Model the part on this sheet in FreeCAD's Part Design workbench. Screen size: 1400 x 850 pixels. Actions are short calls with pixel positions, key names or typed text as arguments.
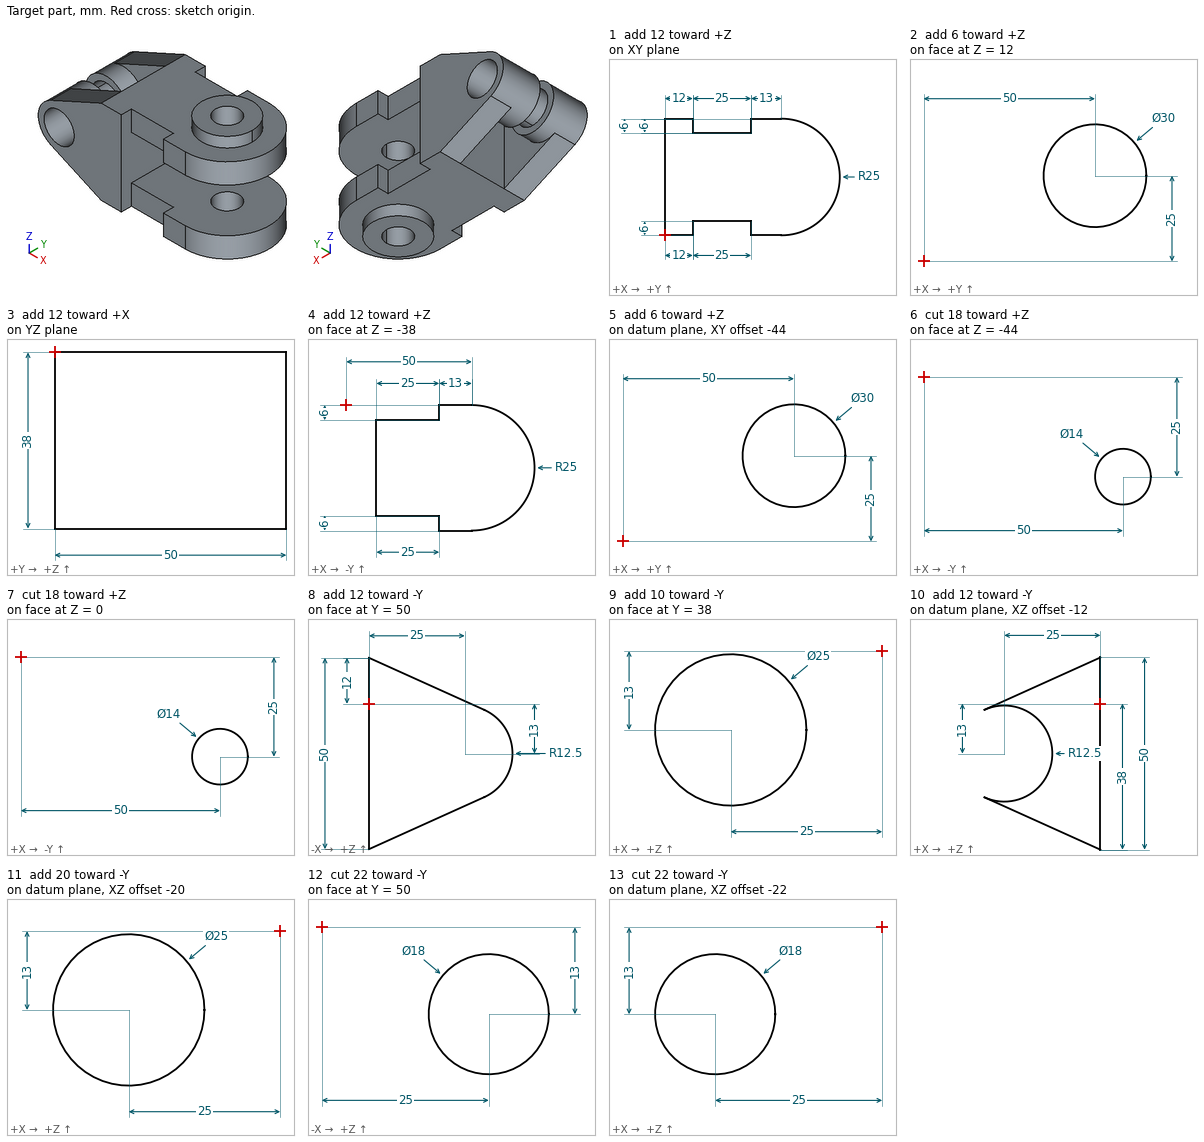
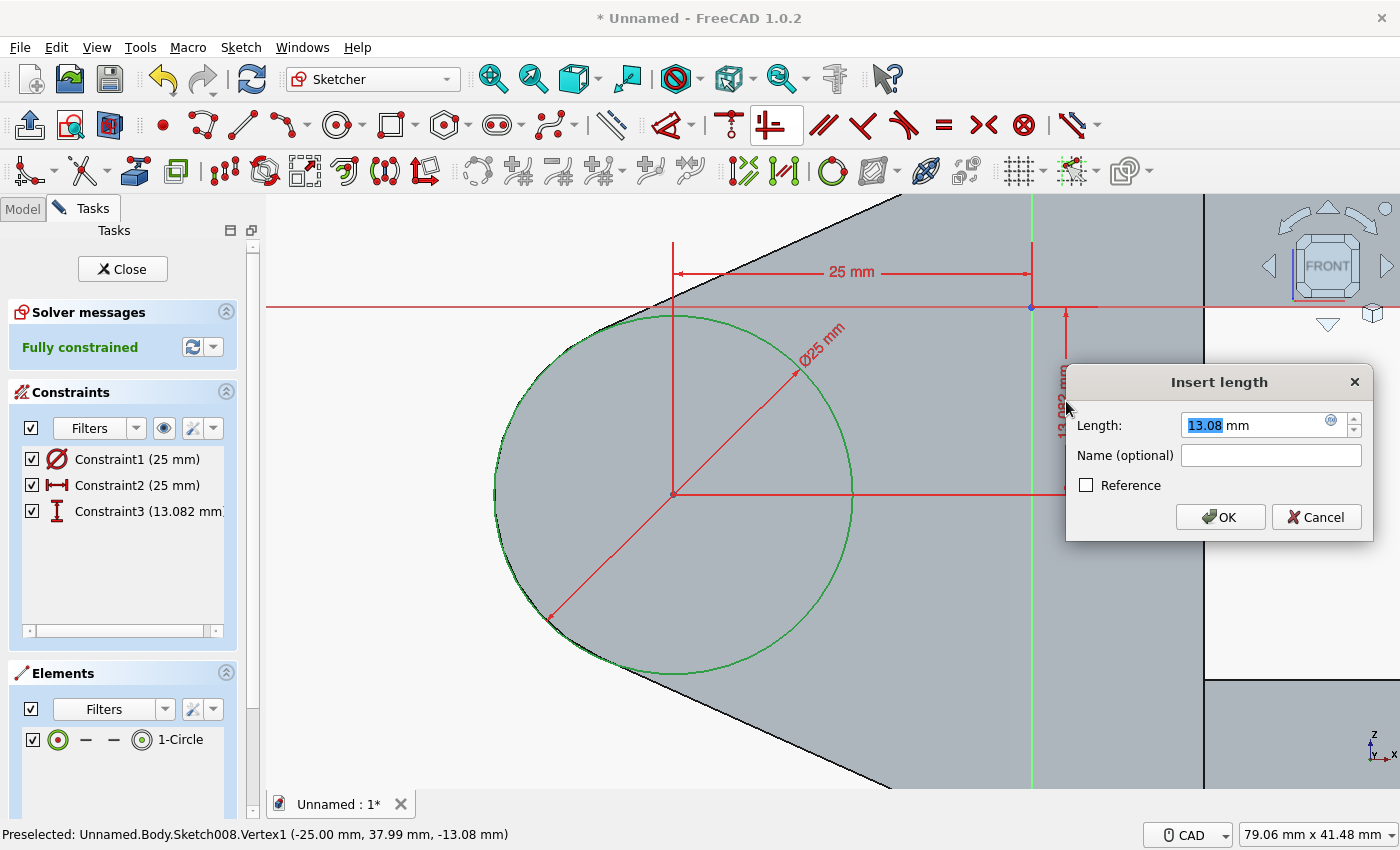
text(13)
key(Return)
key(Escape)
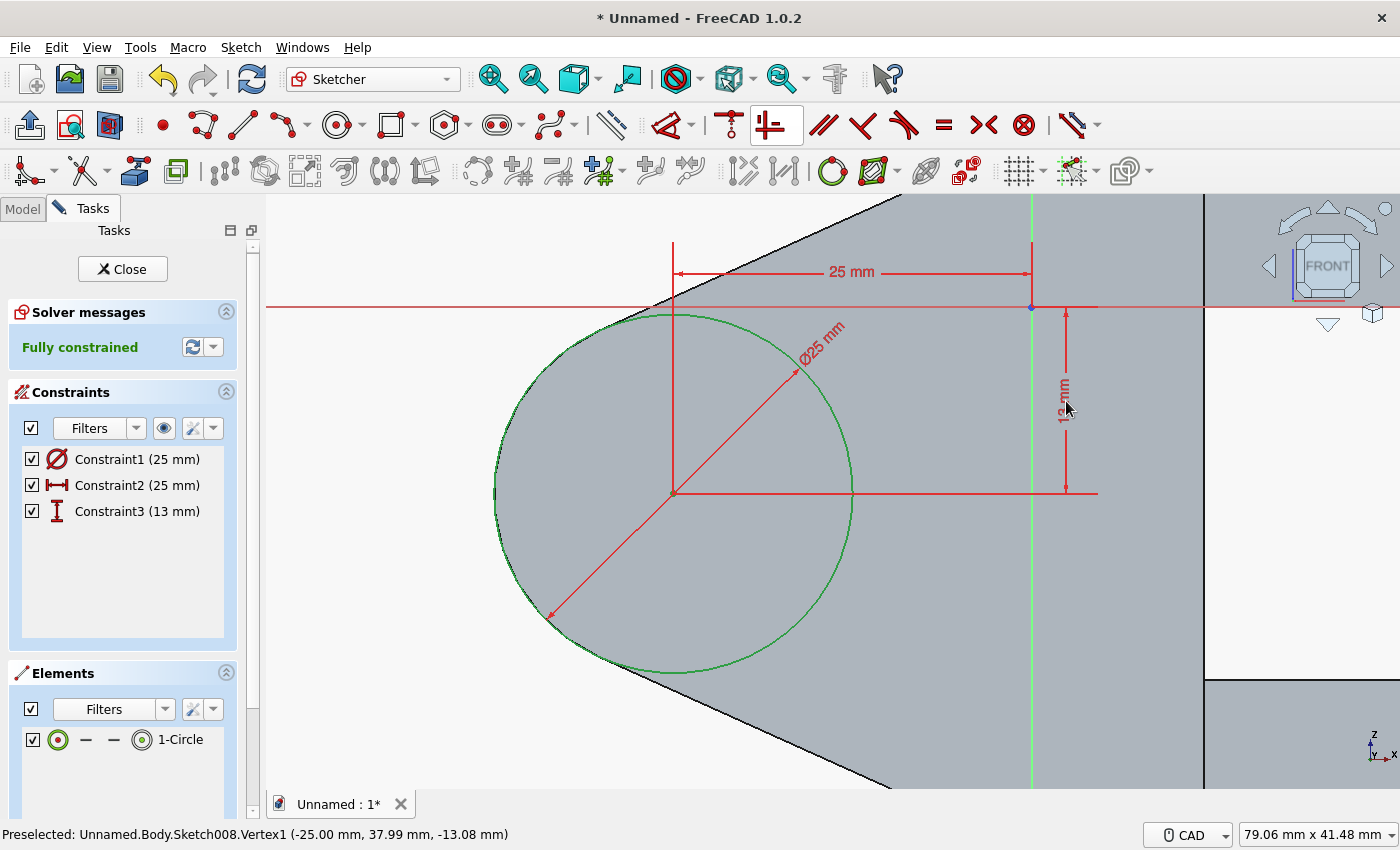
click(123, 269)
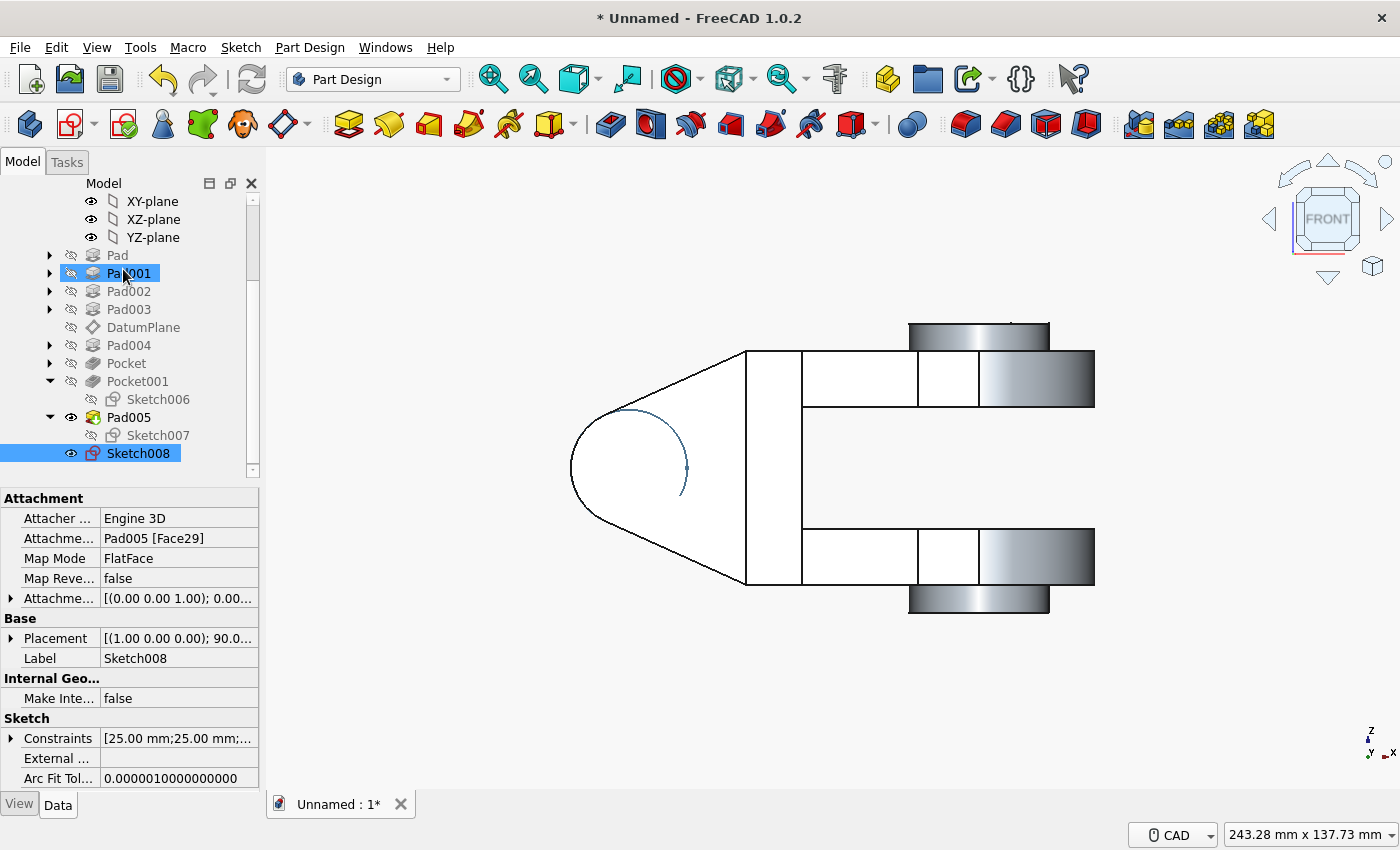
click(350, 124)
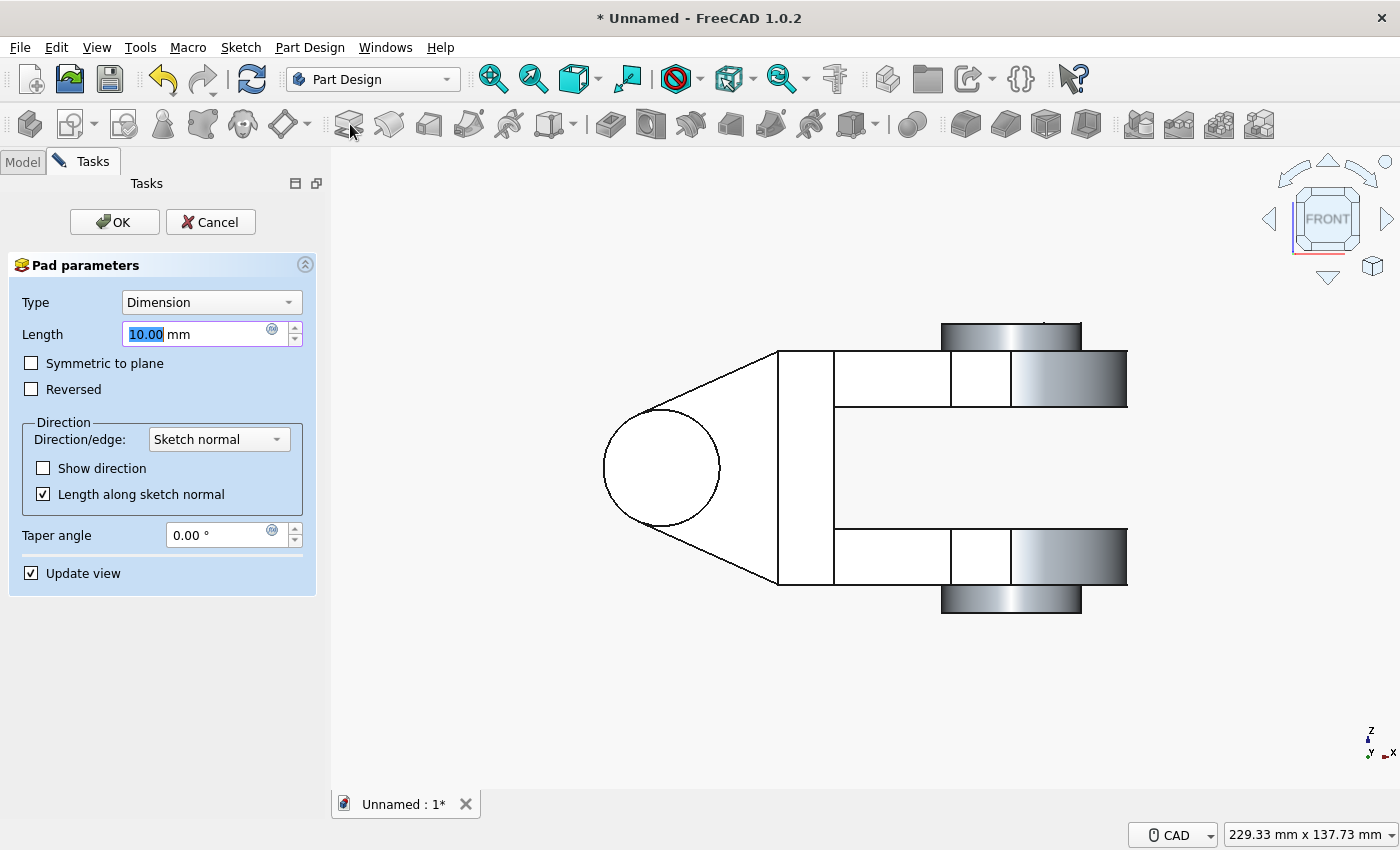
text(10)
key(Tab)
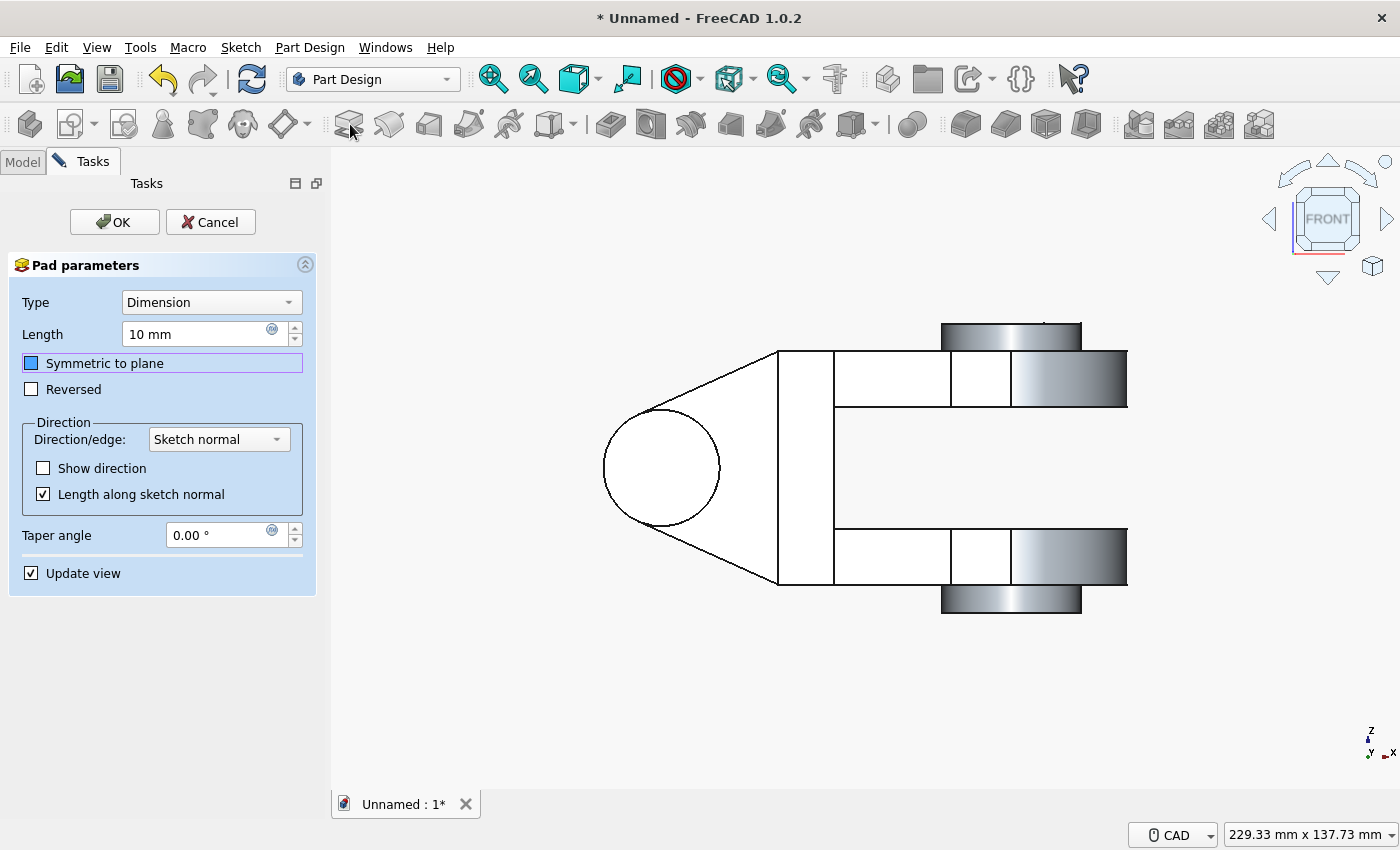
click(115, 222)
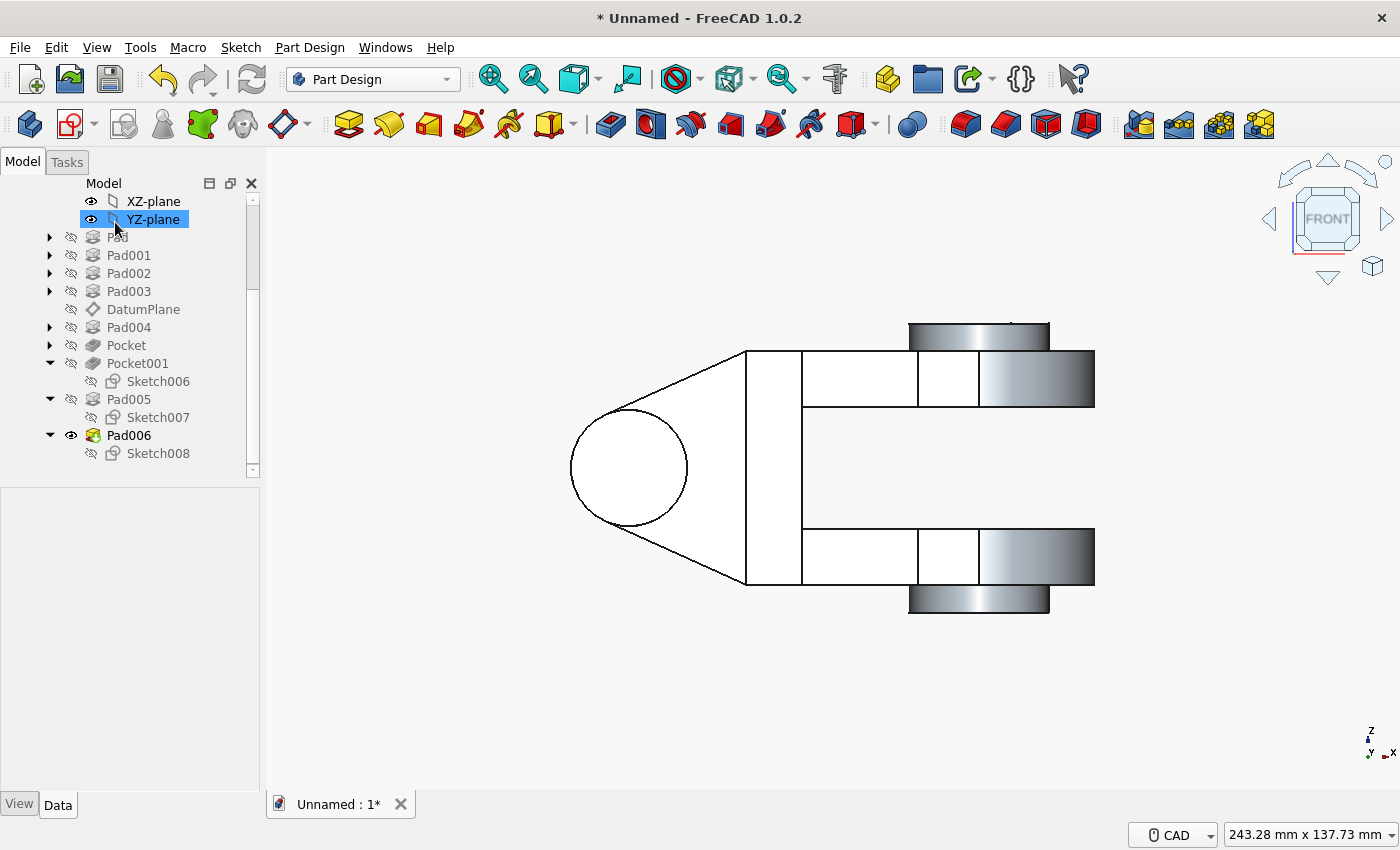
scroll(160, 323, down, 3)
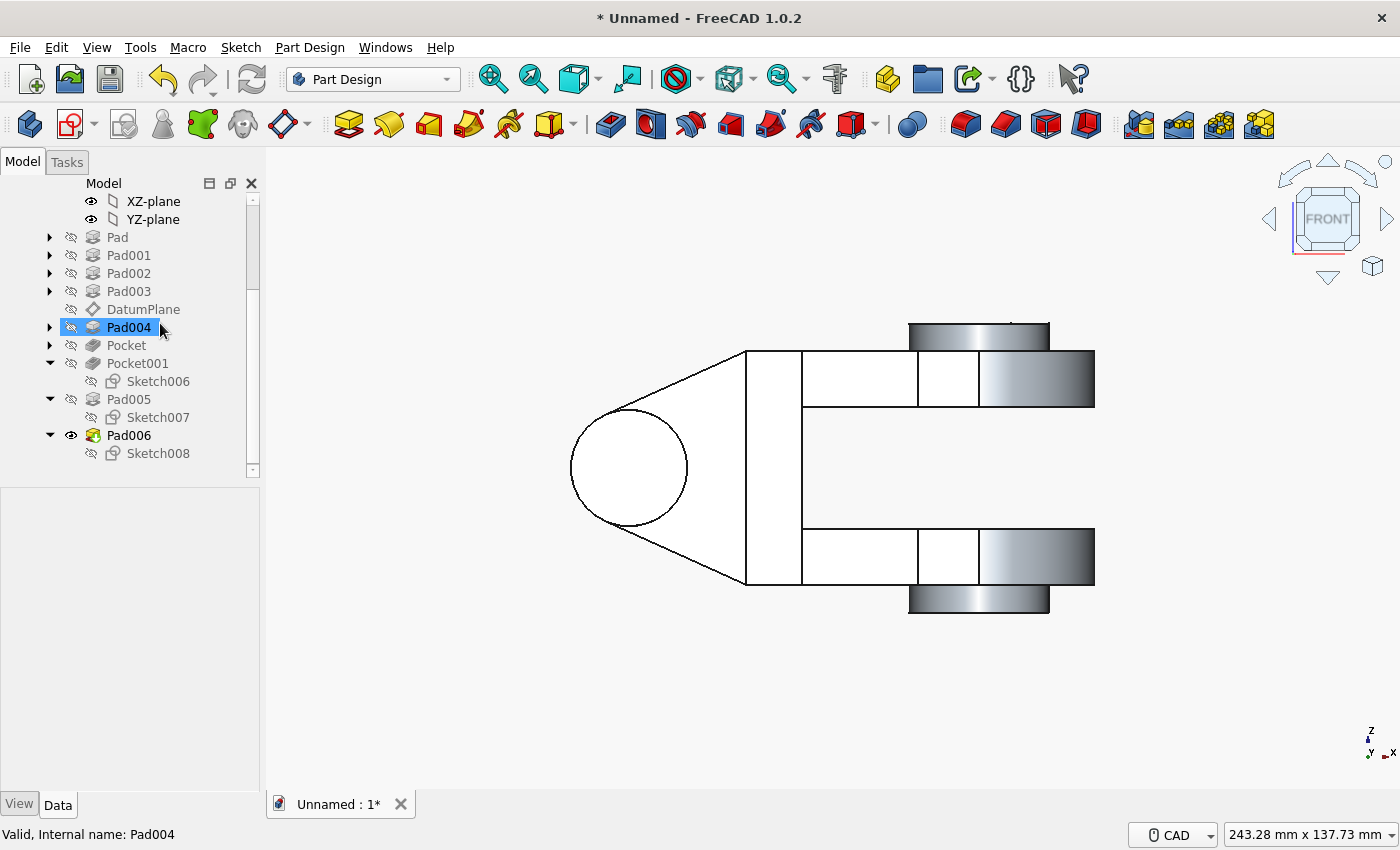
scroll(160, 323, up, 15)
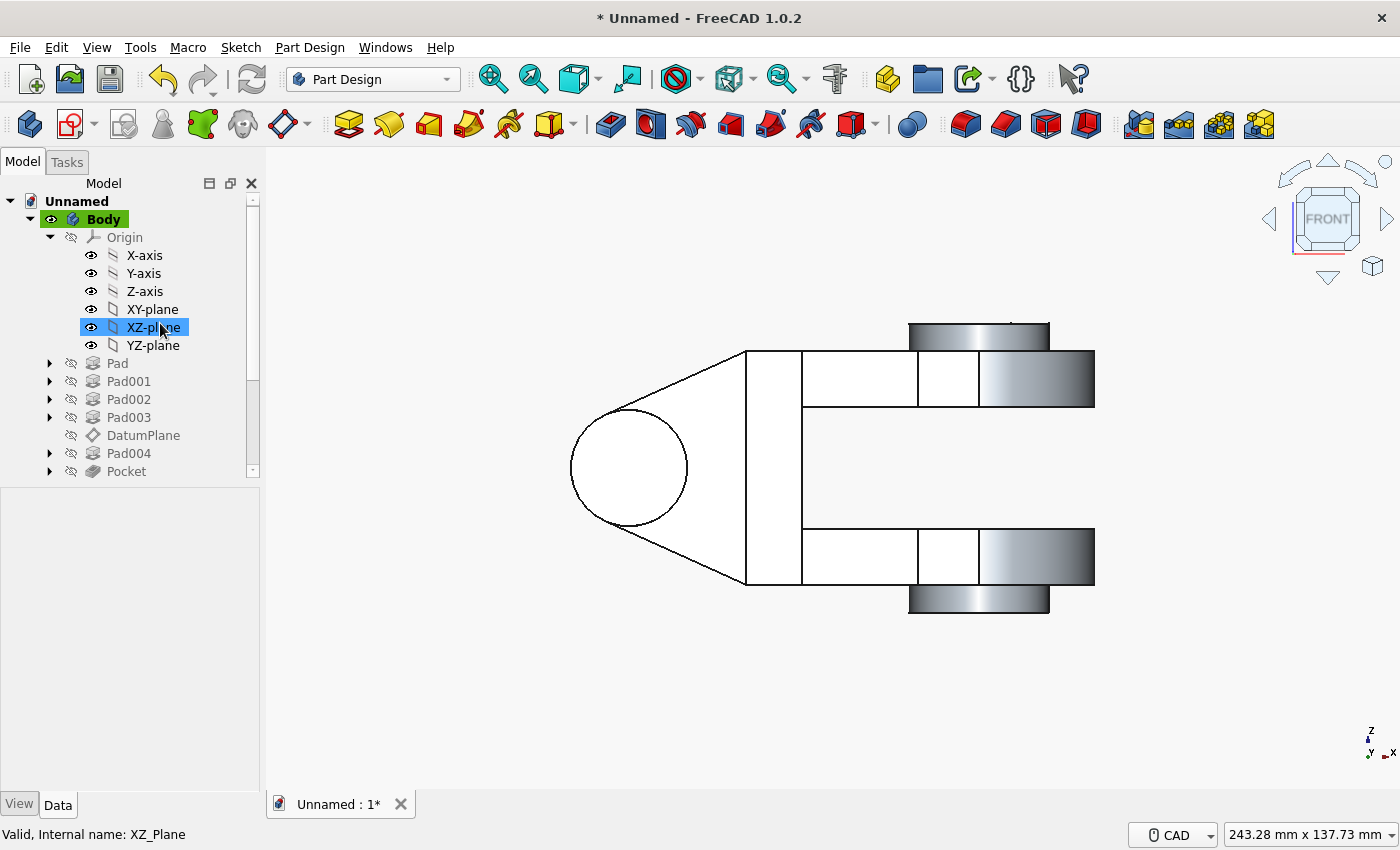
click(136, 327)